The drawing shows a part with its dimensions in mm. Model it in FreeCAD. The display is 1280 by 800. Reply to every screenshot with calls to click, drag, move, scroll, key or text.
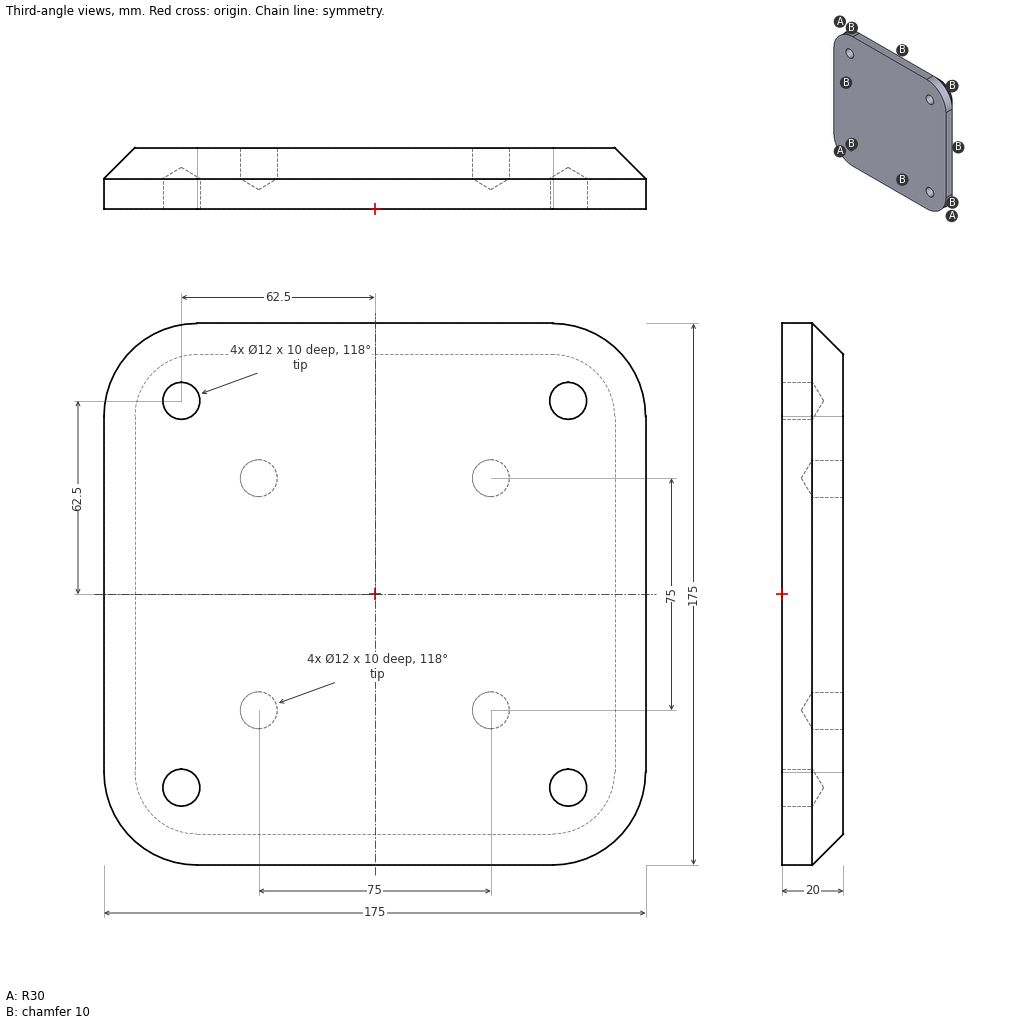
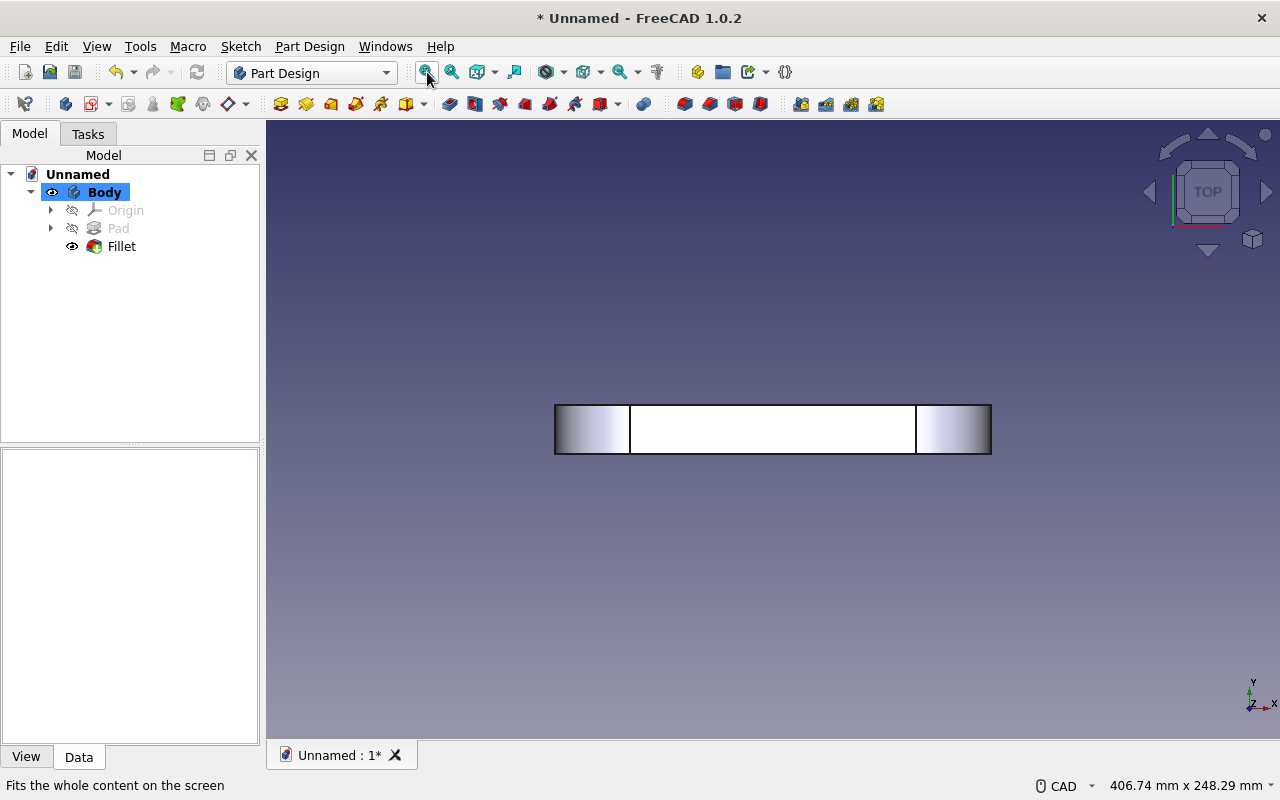
key(1)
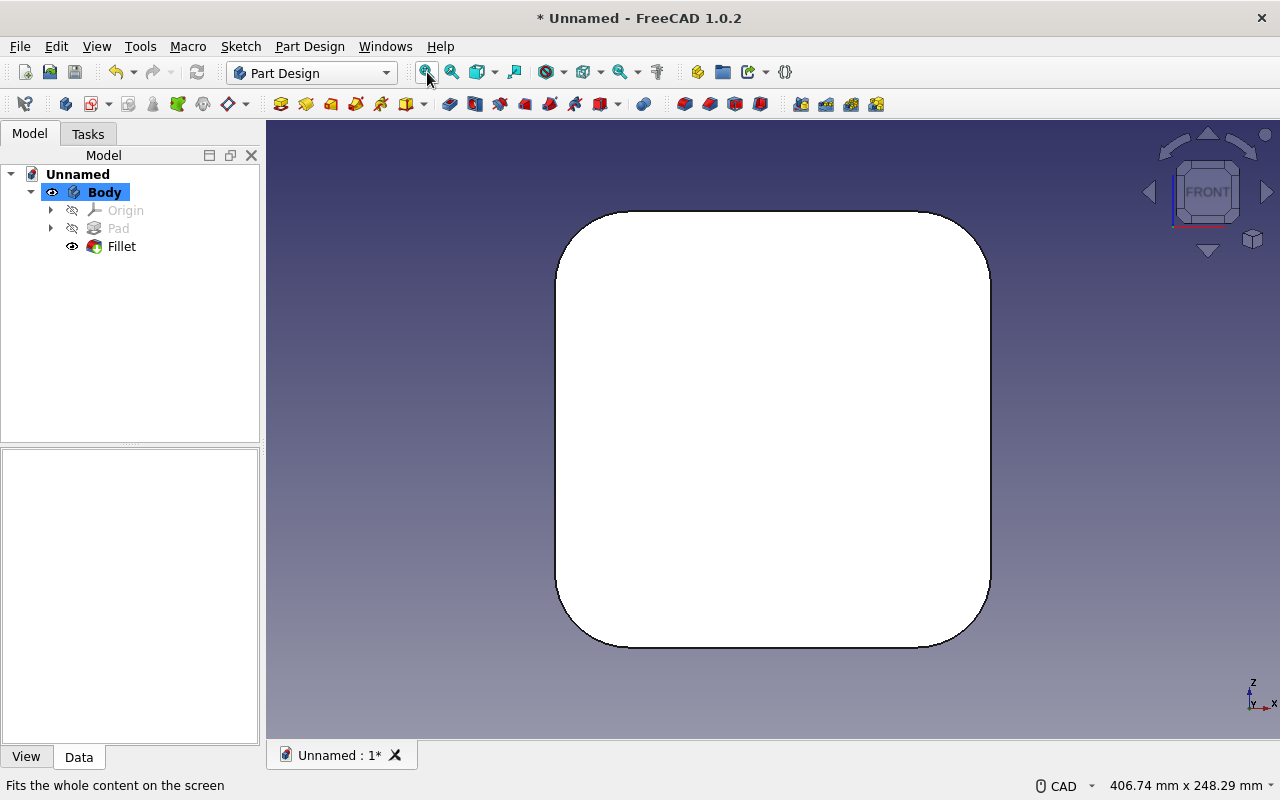
key(3)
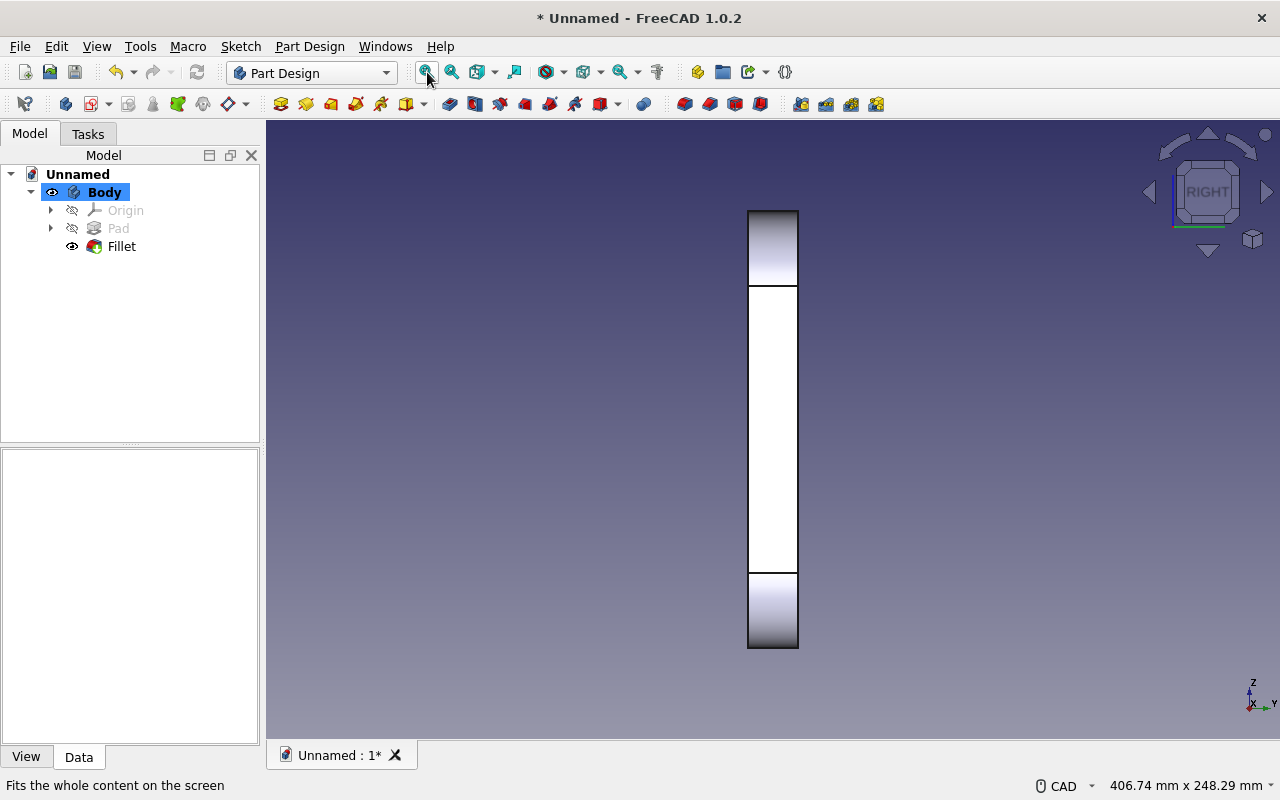
key(5)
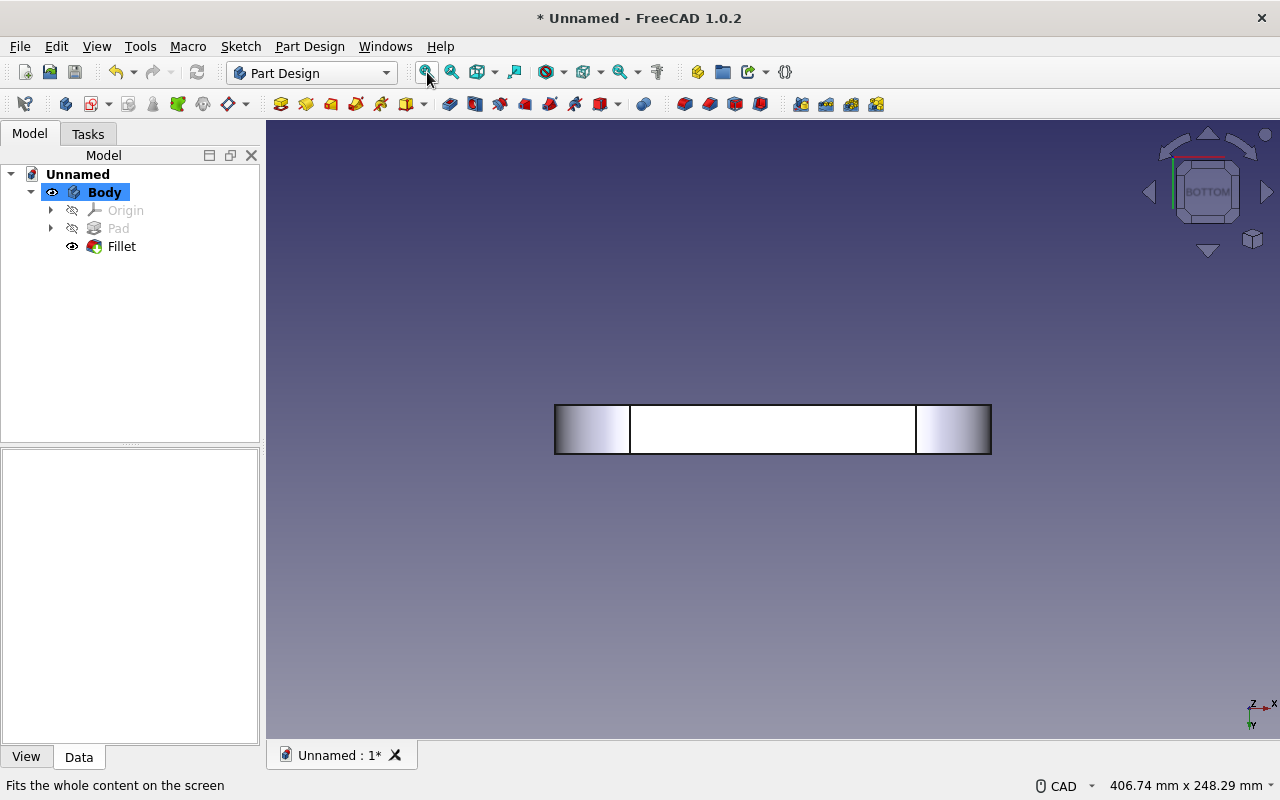
click(427, 72)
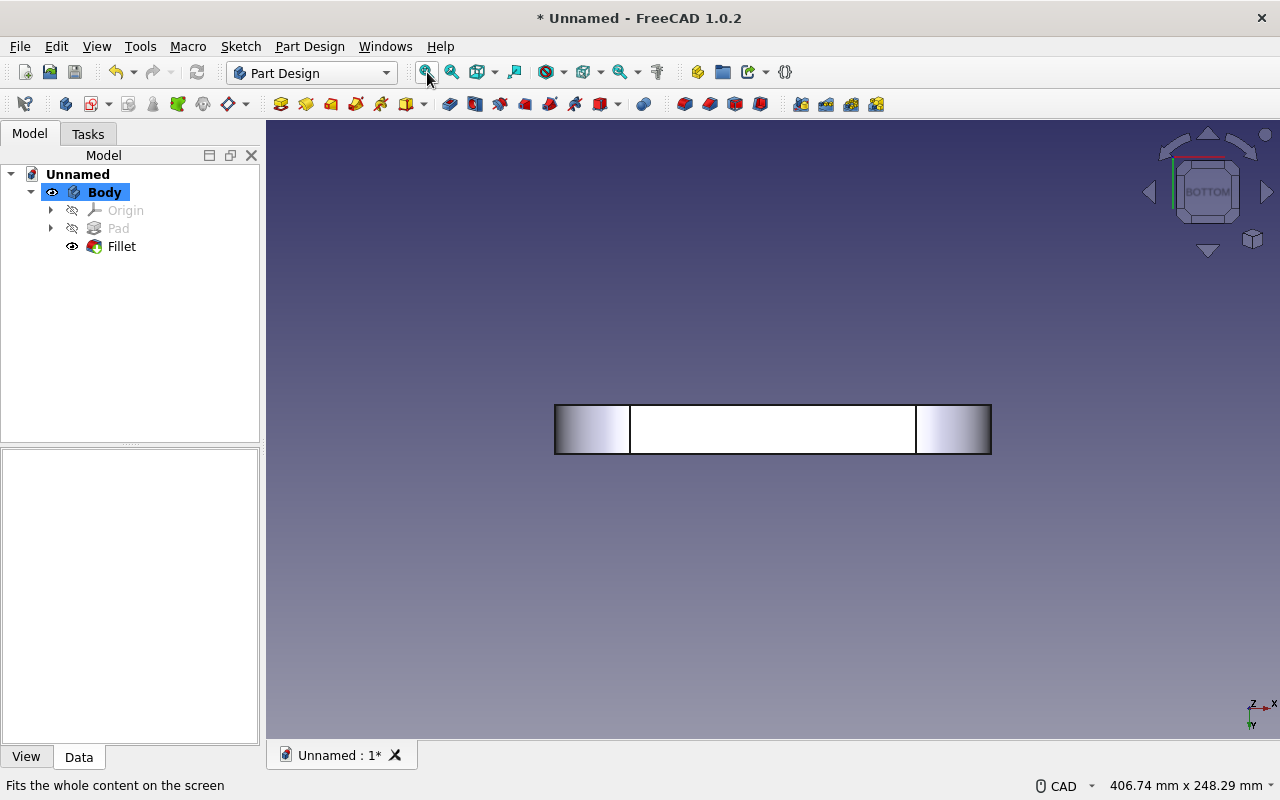
key(4)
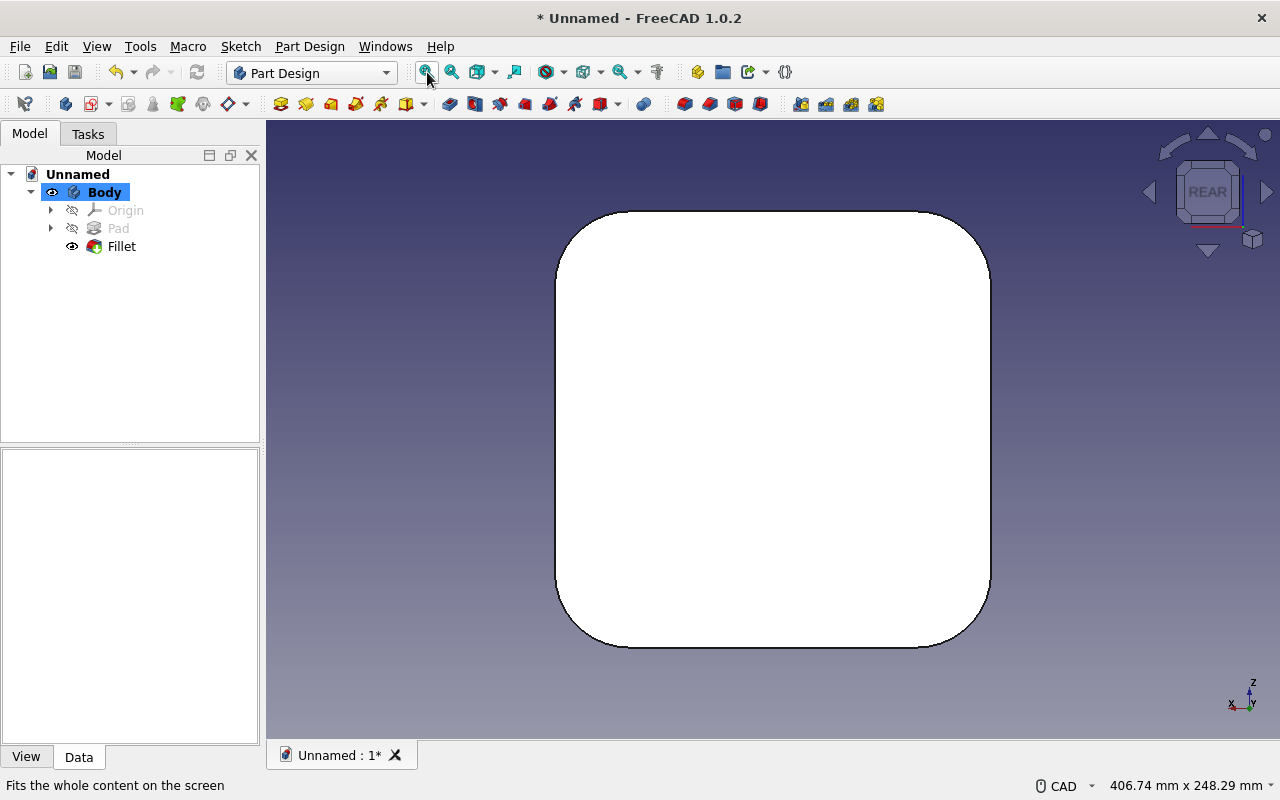
click(773, 429)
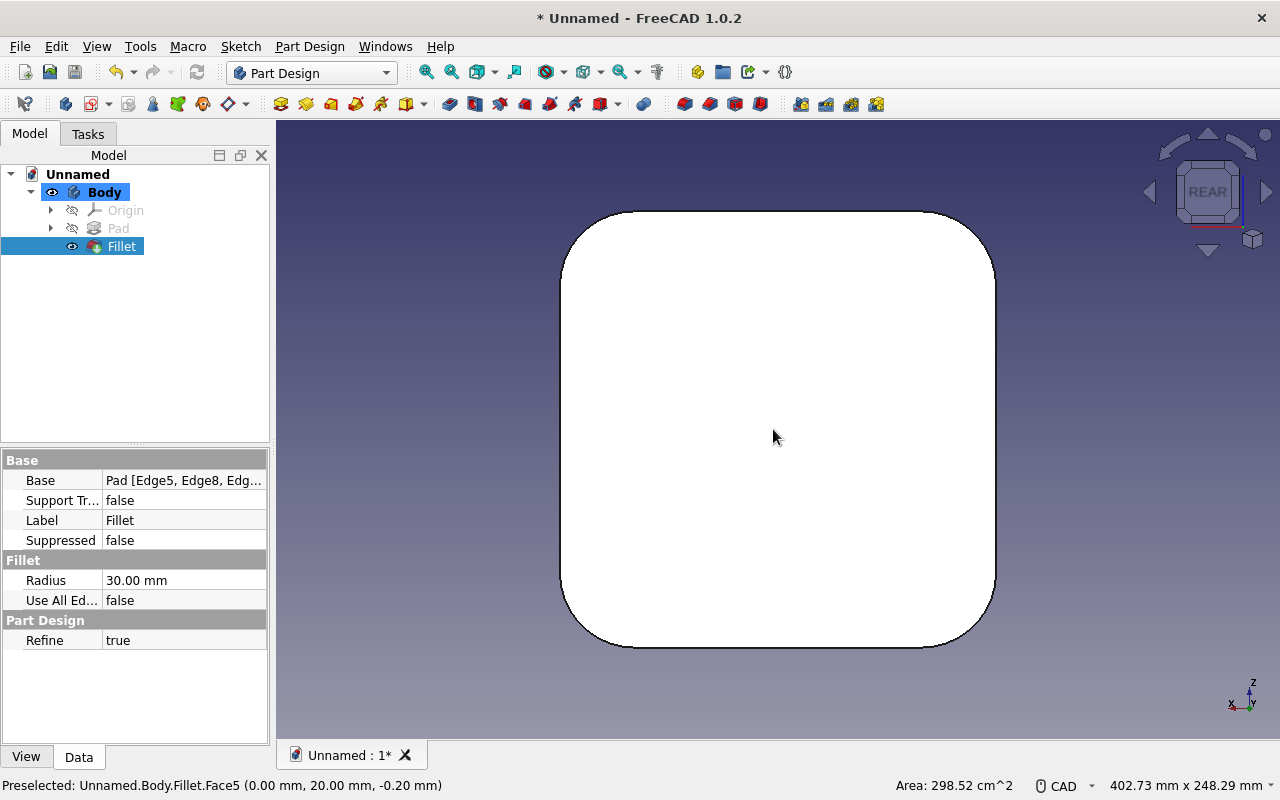
click(710, 104)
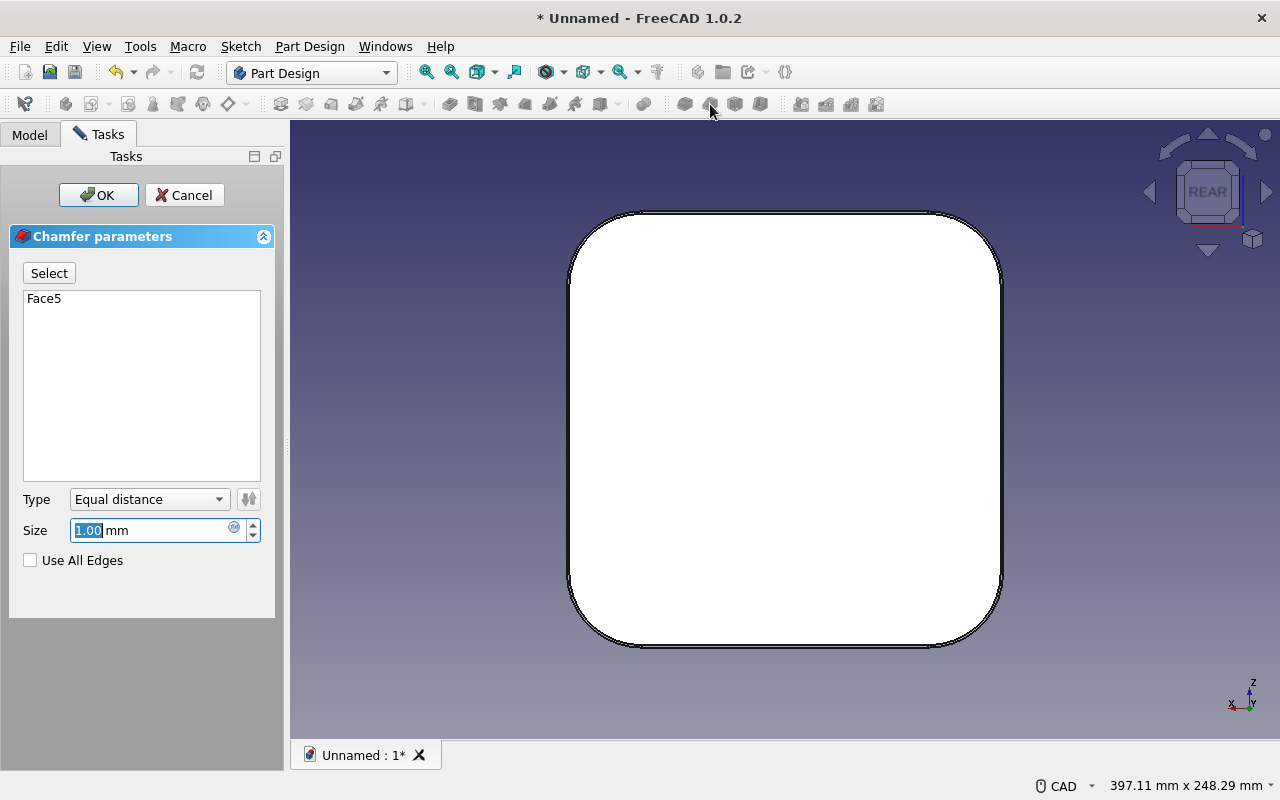
text(10)
key(Tab)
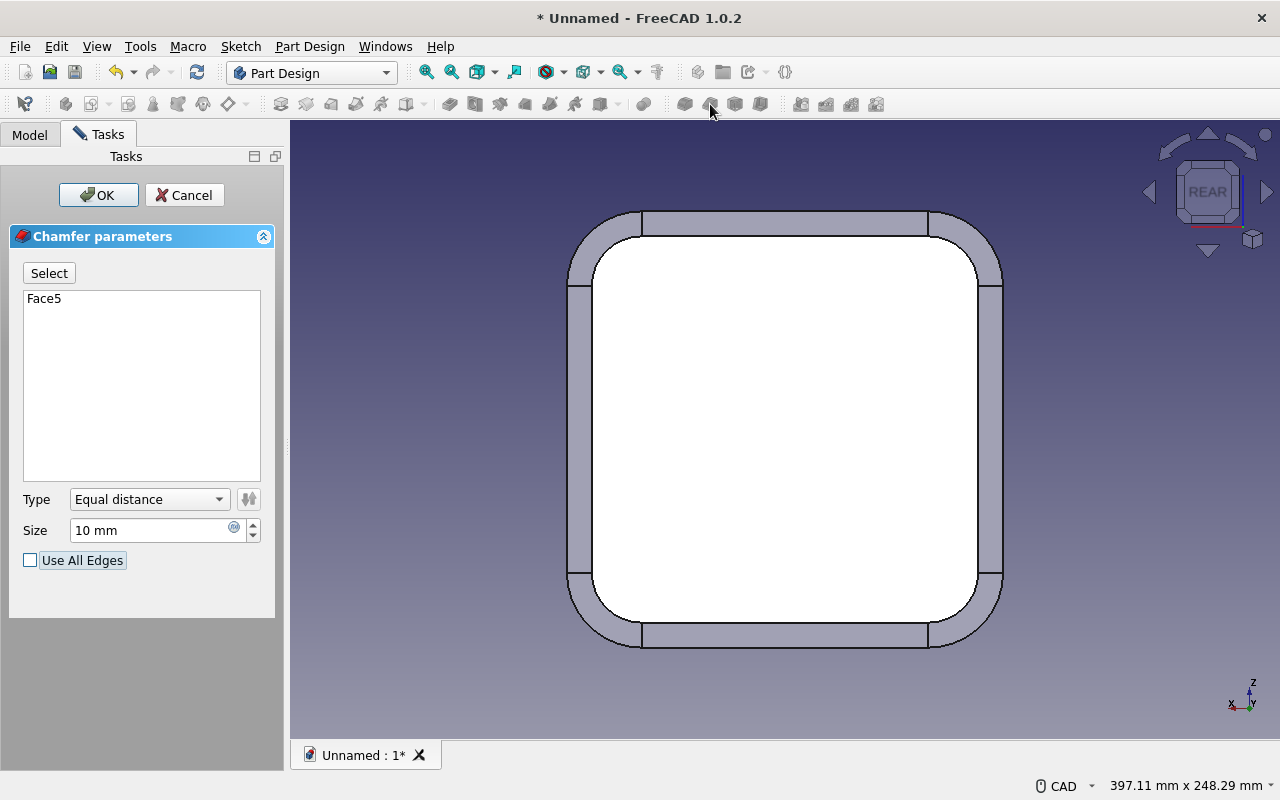
click(99, 195)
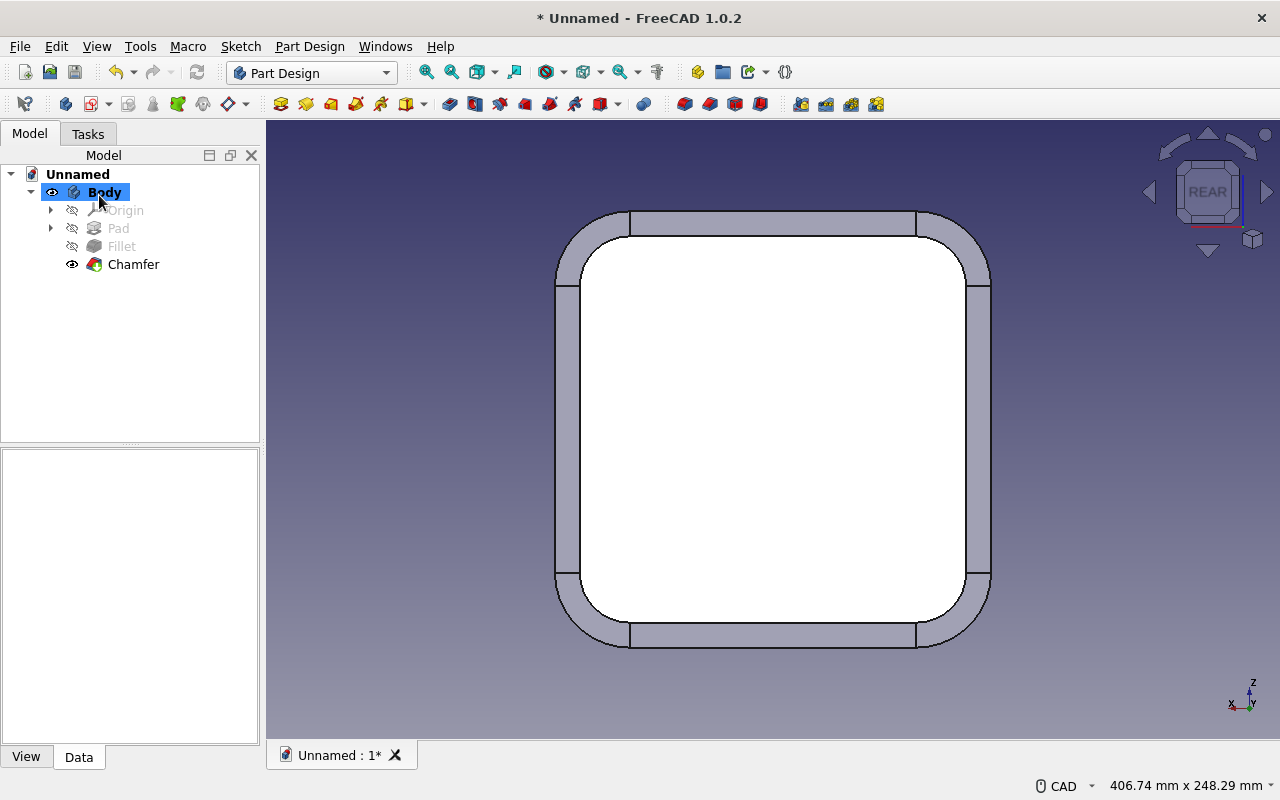
click(773, 429)